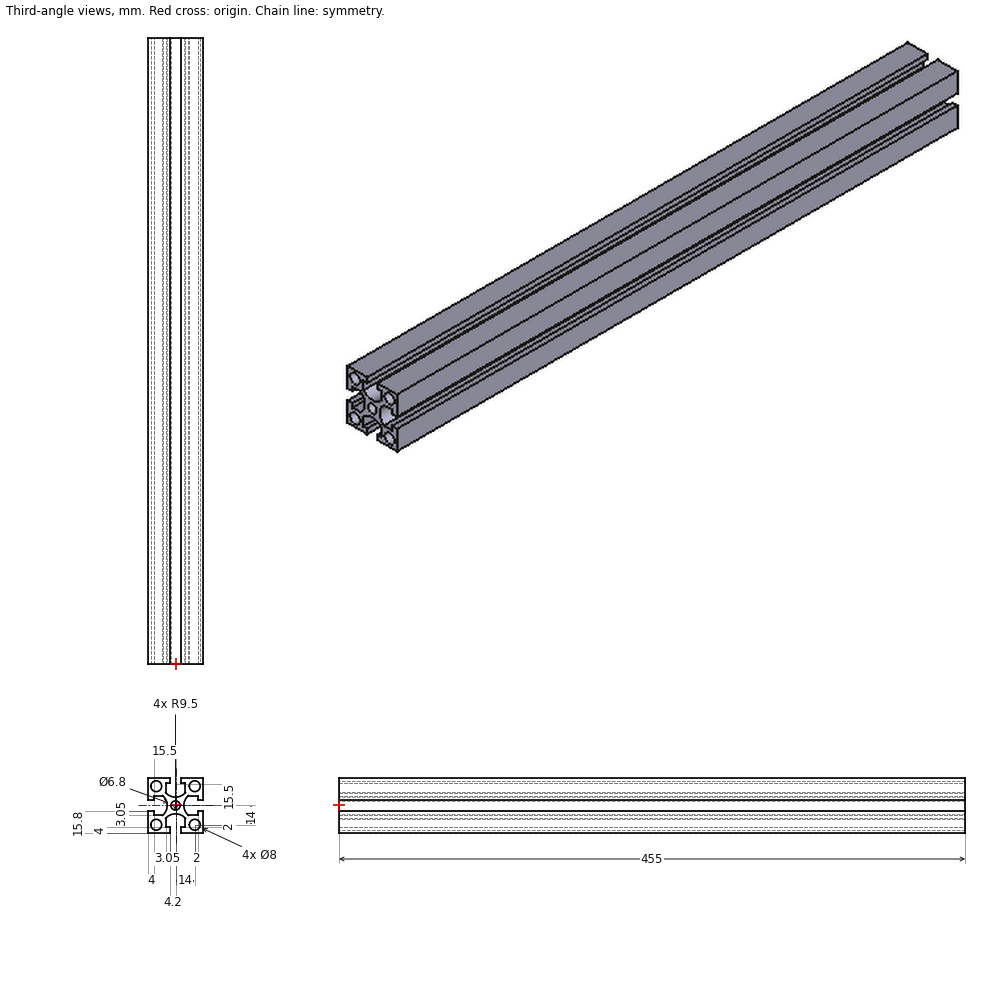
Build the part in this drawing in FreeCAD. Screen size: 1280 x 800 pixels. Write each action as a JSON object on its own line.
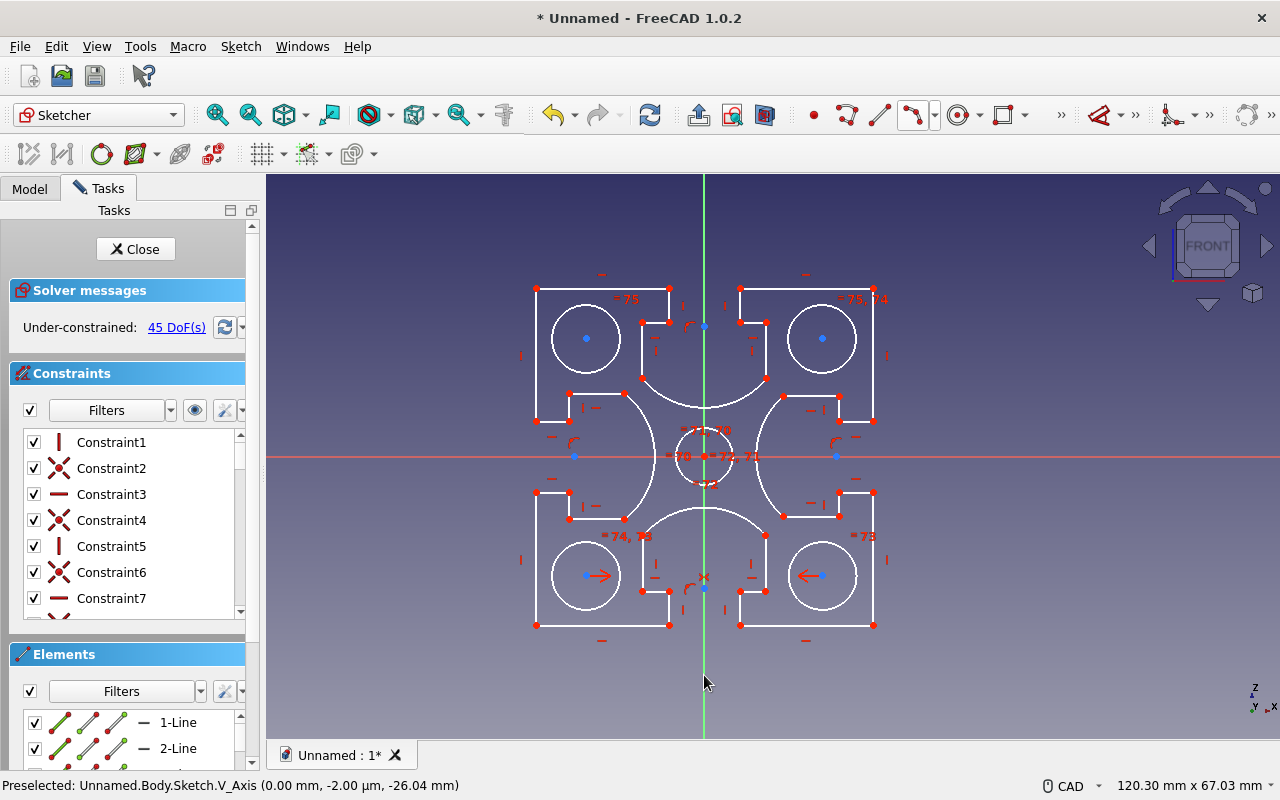
{"action": "left_click", "coordinate": [823, 576]}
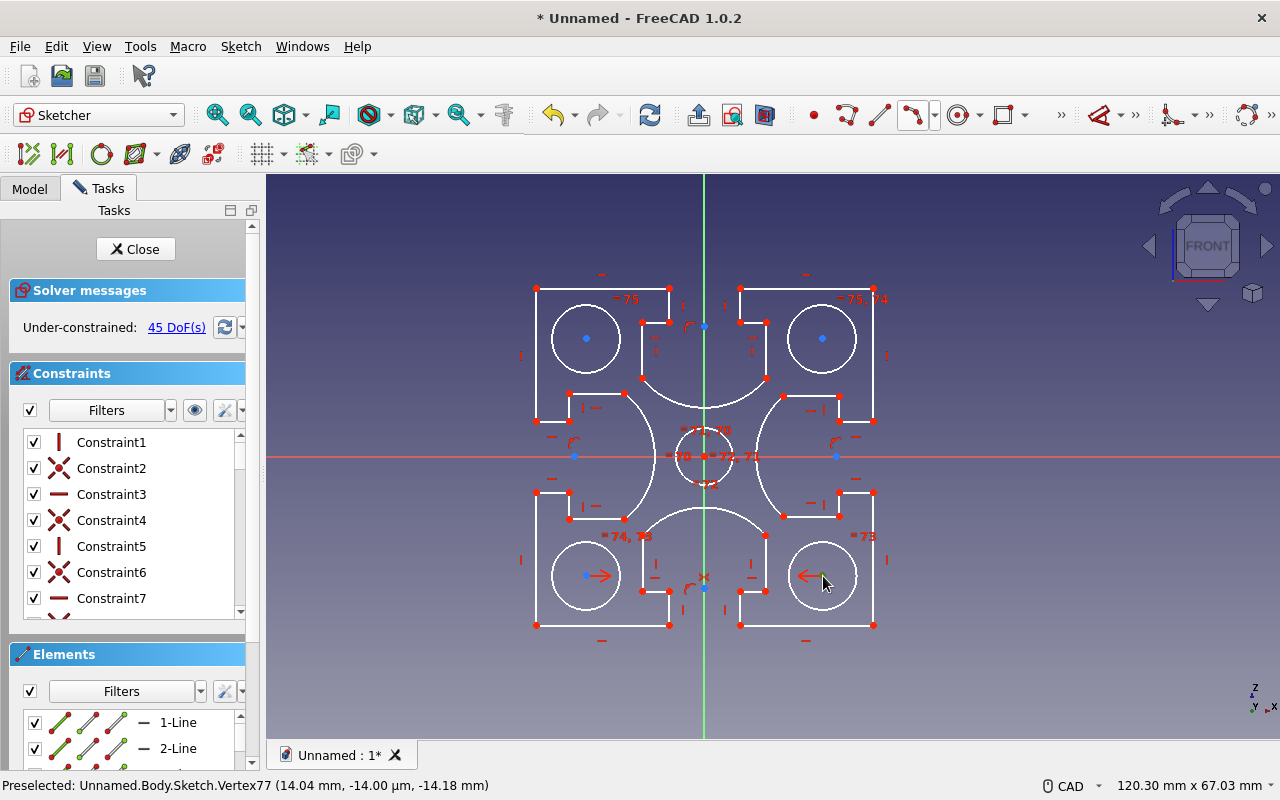
{"action": "left_click", "coordinate": [822, 339]}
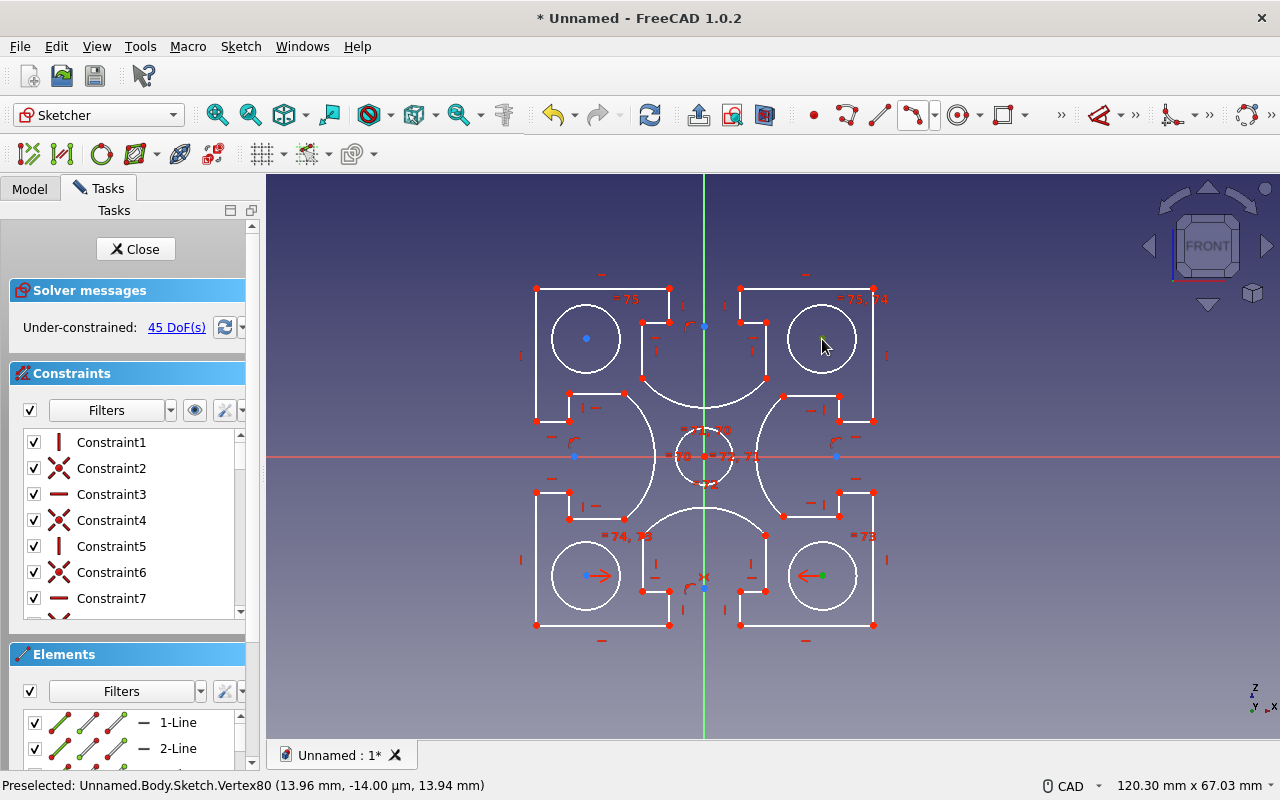
{"action": "left_click", "coordinate": [353, 456]}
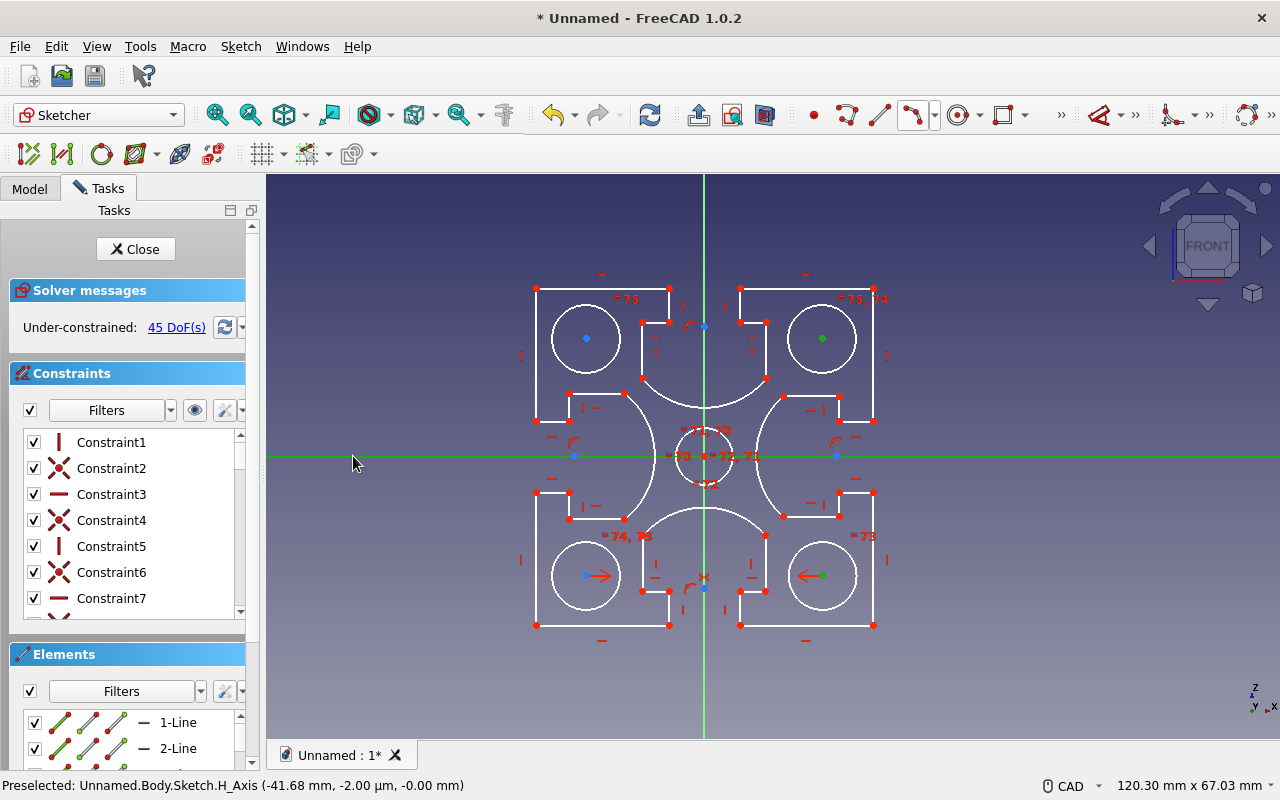
{"action": "key", "text": "s"}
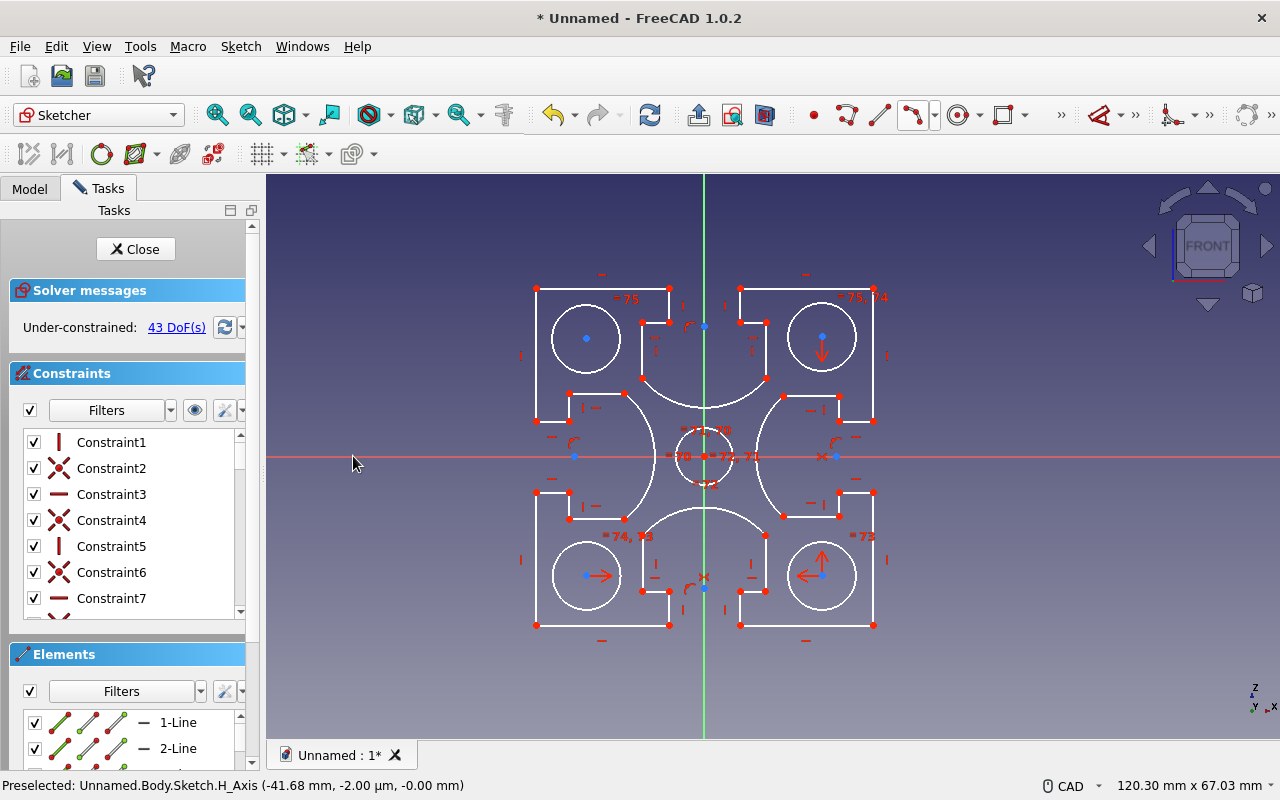
{"action": "left_click", "coordinate": [822, 337]}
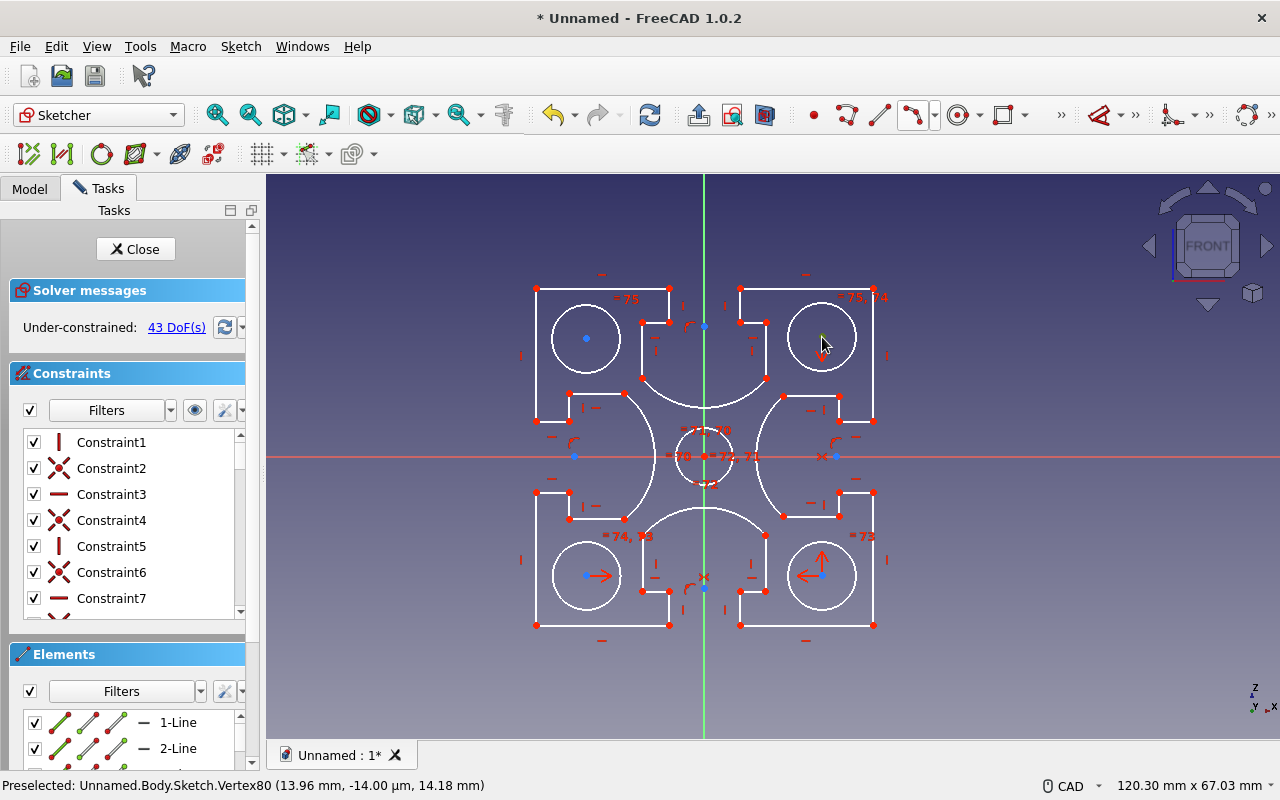
{"action": "left_click", "coordinate": [586, 339]}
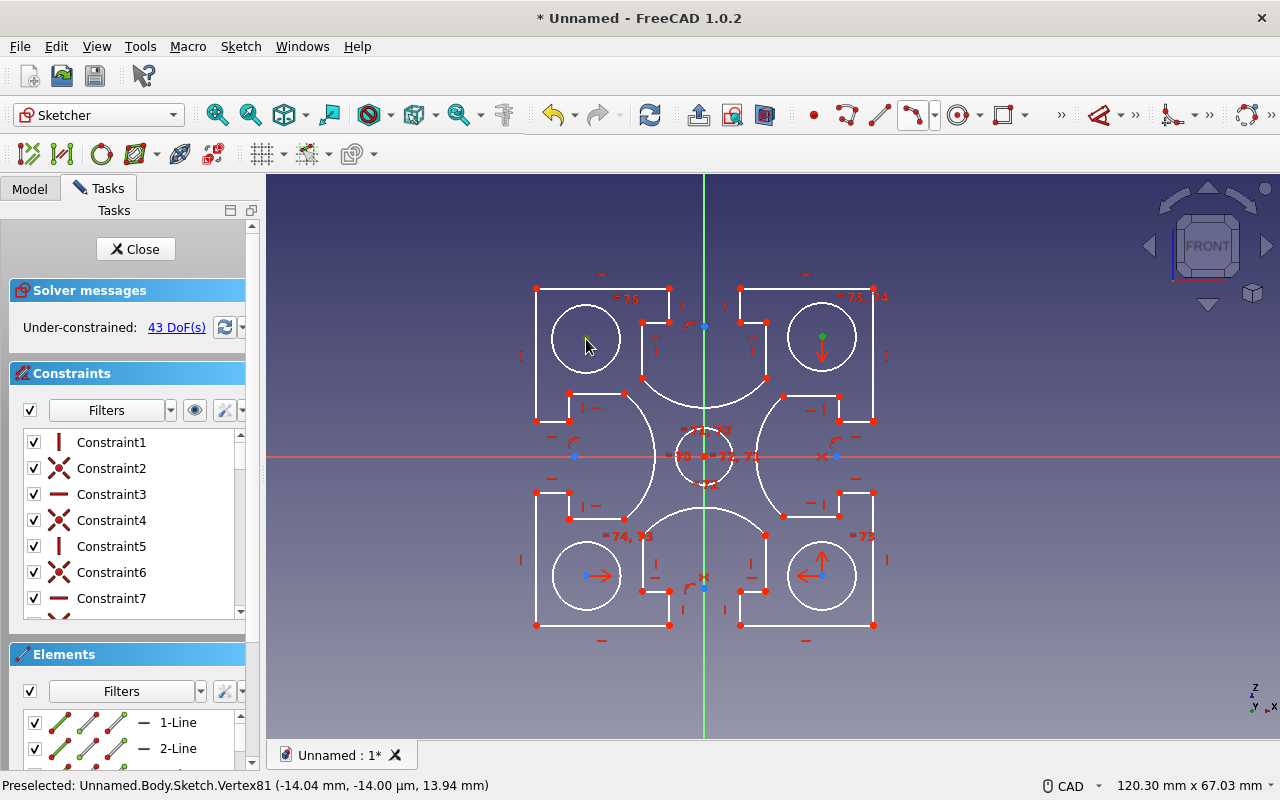
{"action": "left_click", "coordinate": [704, 675]}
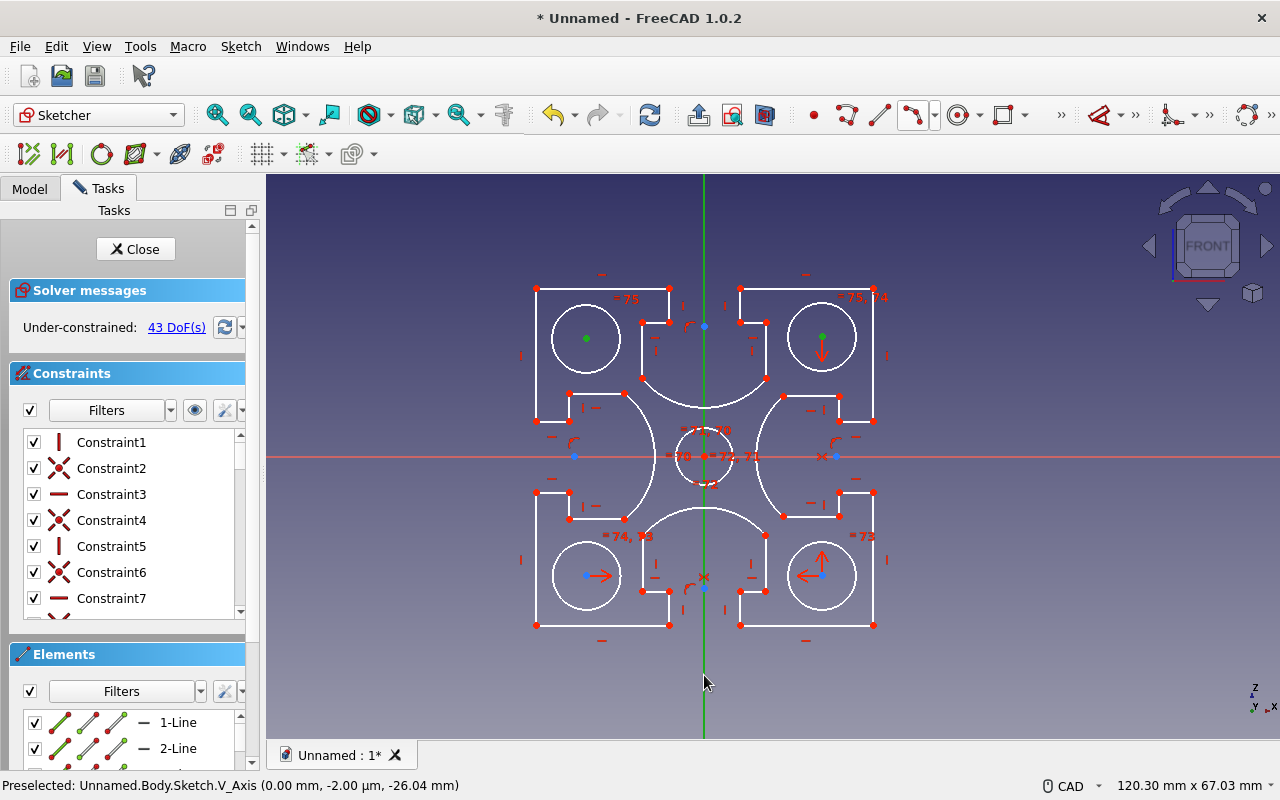
{"action": "key", "text": "s"}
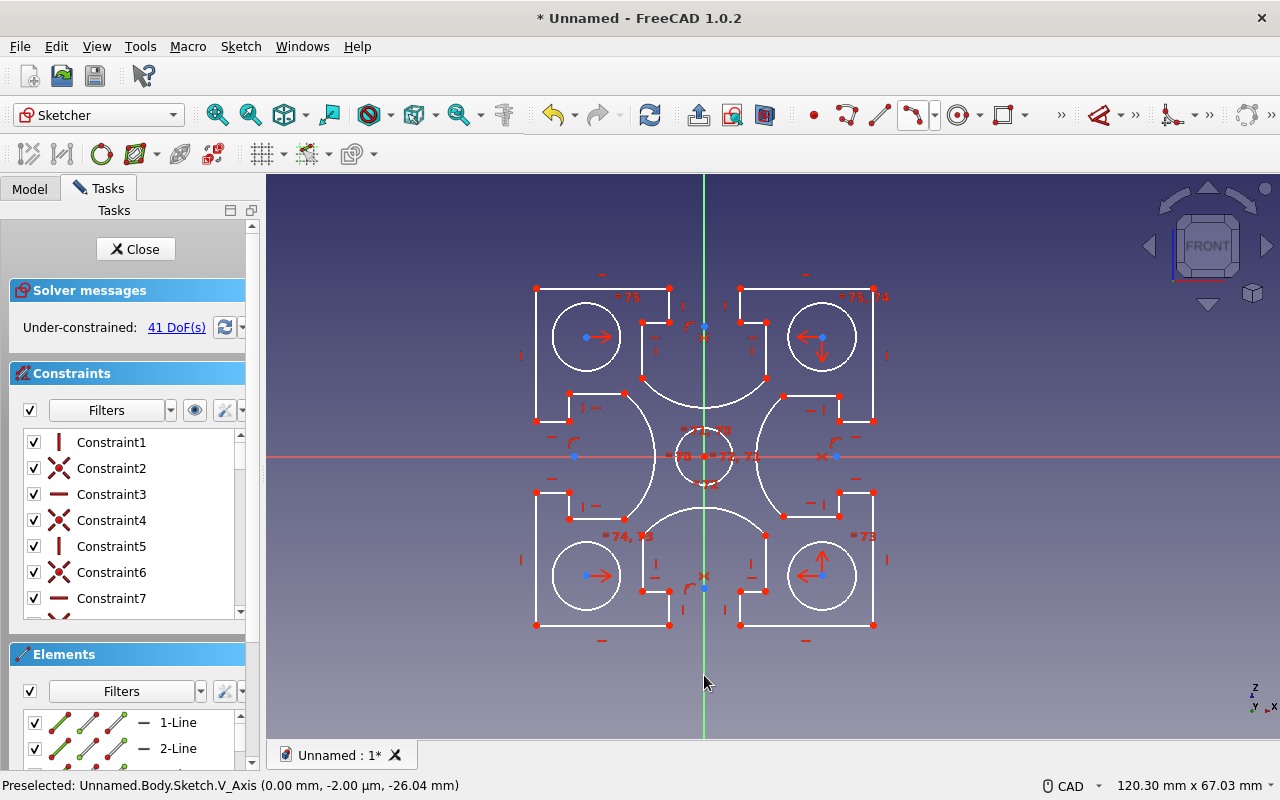
{"action": "left_click", "coordinate": [569, 519]}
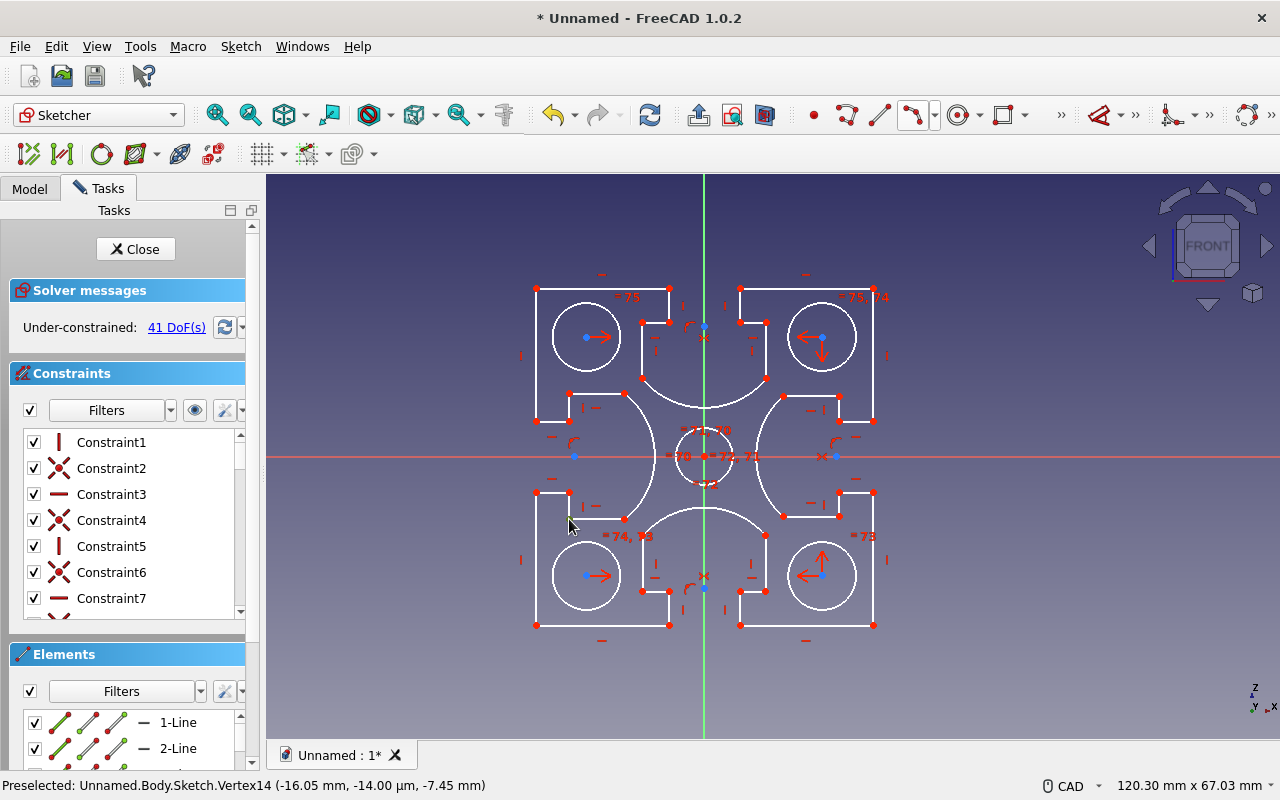
{"action": "left_click", "coordinate": [569, 394]}